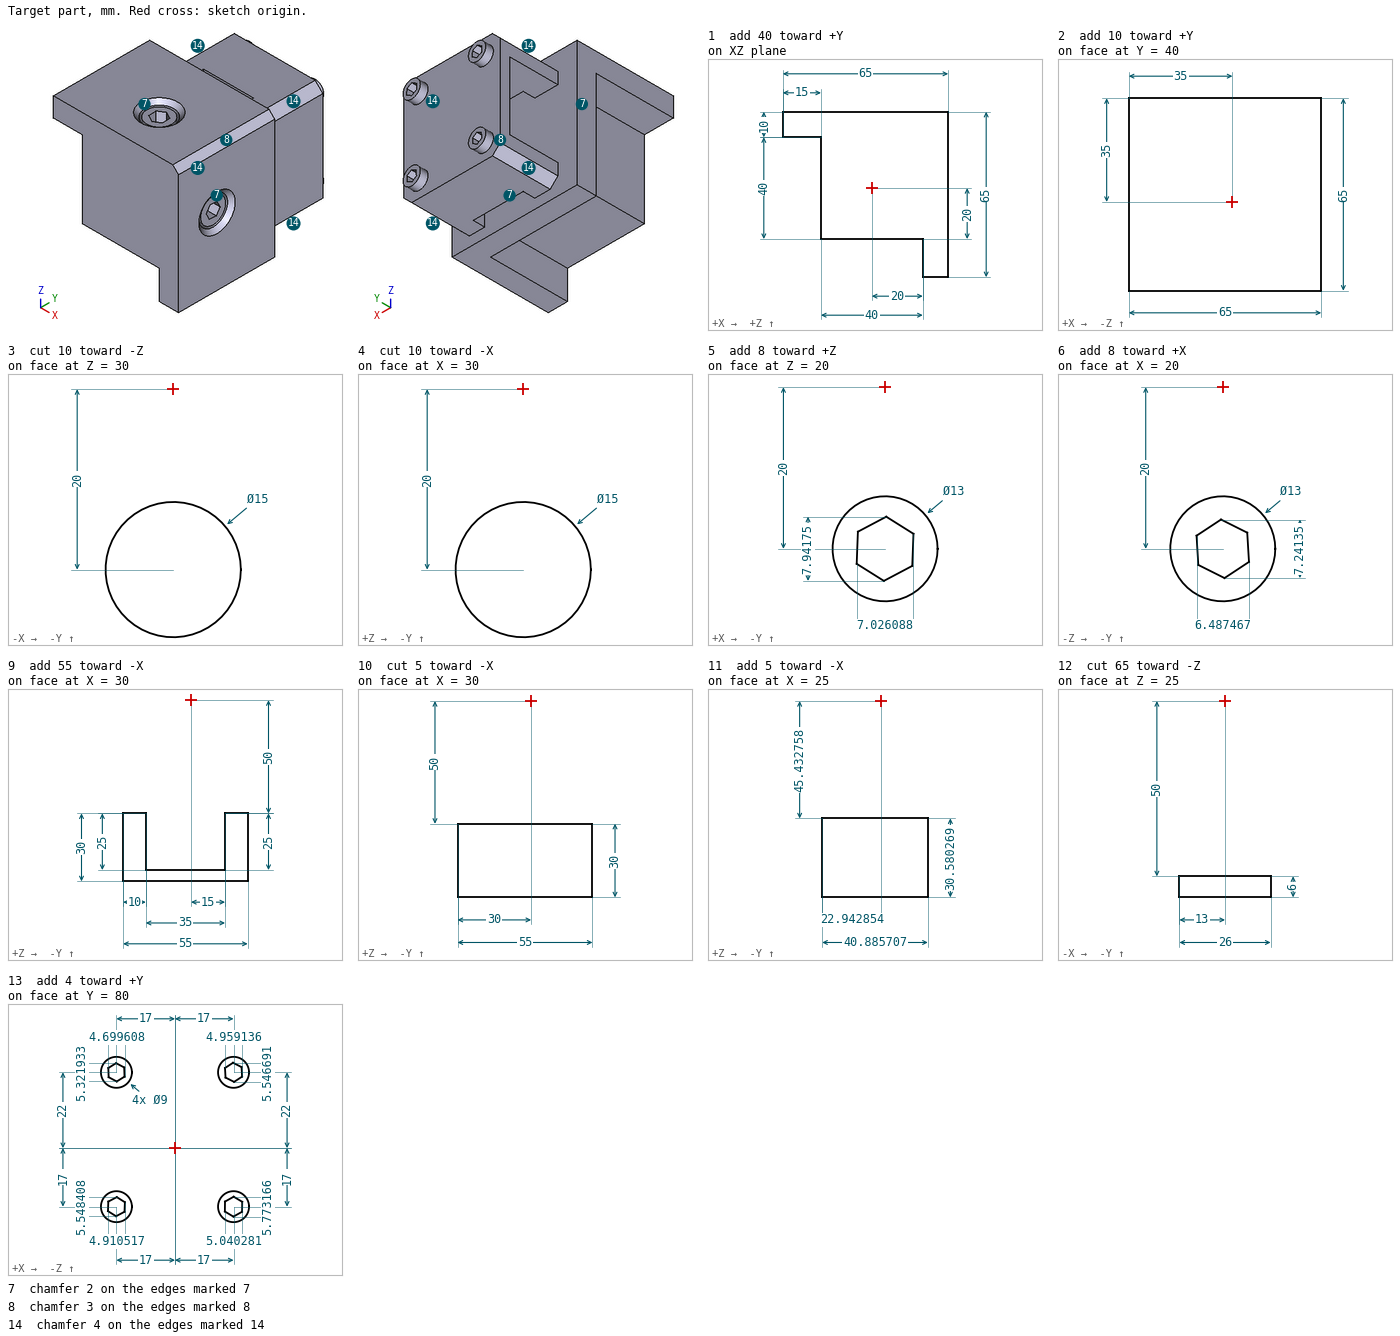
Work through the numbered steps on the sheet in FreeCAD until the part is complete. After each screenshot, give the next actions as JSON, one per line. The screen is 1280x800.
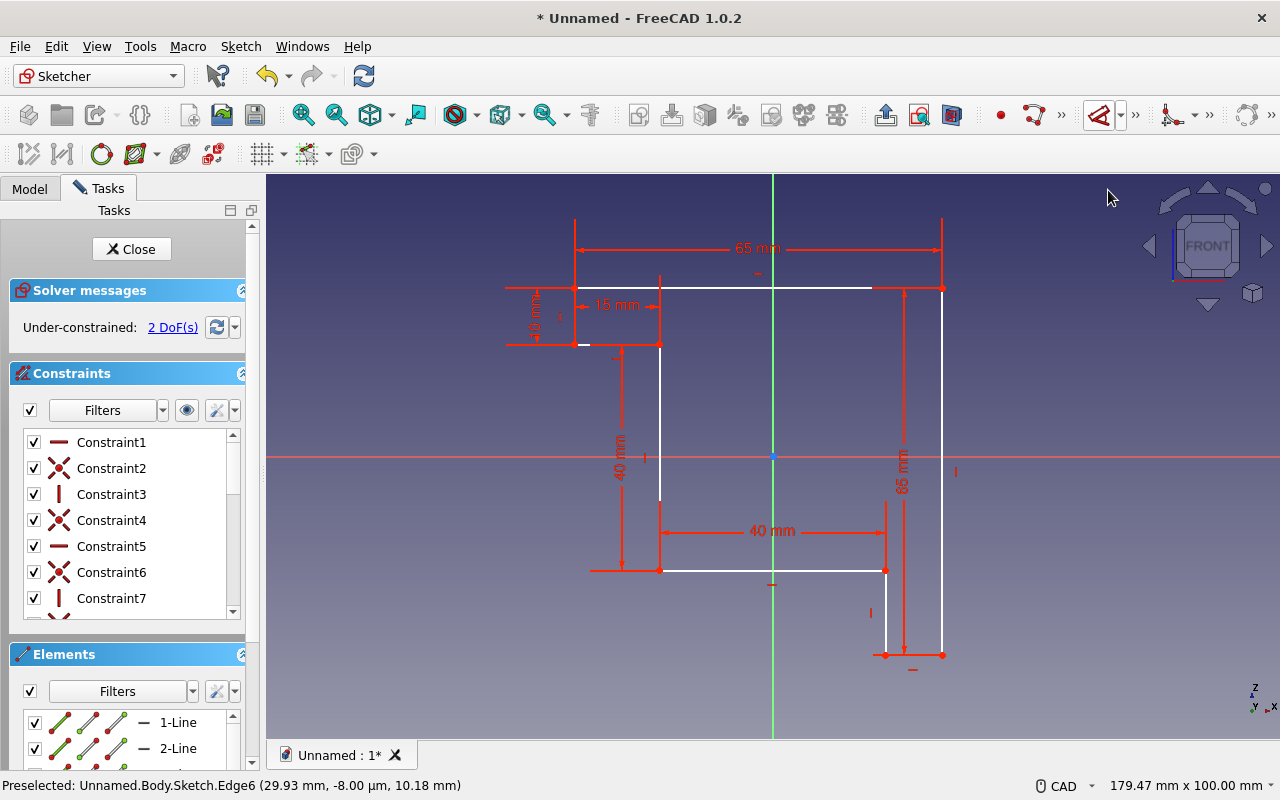
{"action": "left_click", "coordinate": [886, 571]}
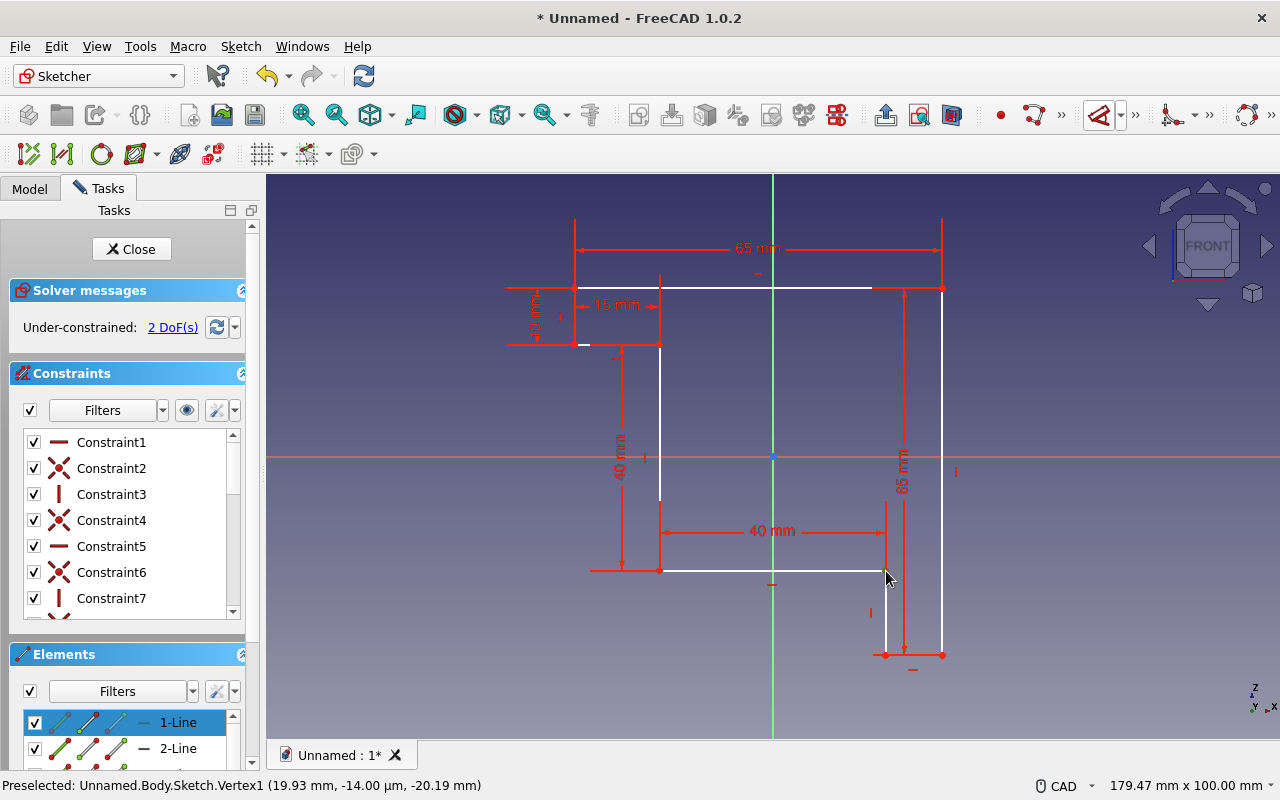
{"action": "key", "text": "l"}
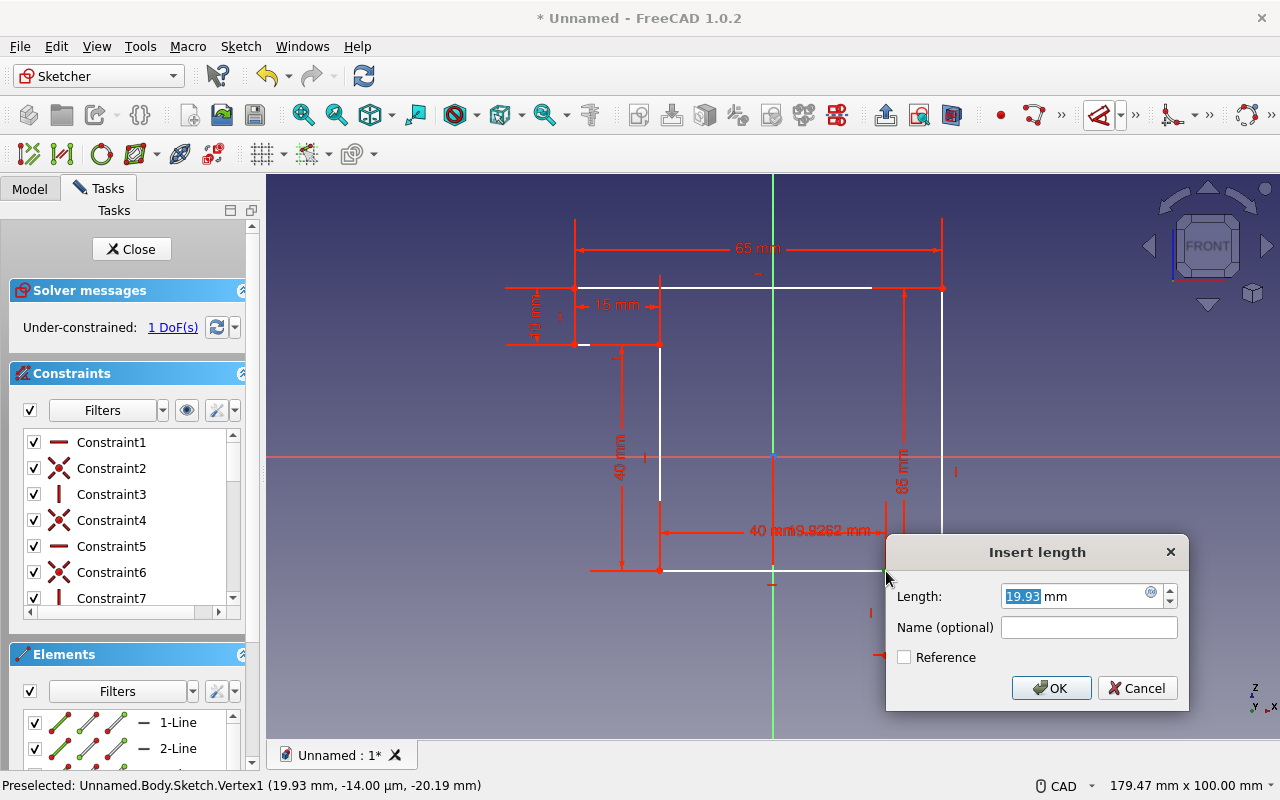
{"action": "type", "text": "20"}
{"action": "key", "text": "Return"}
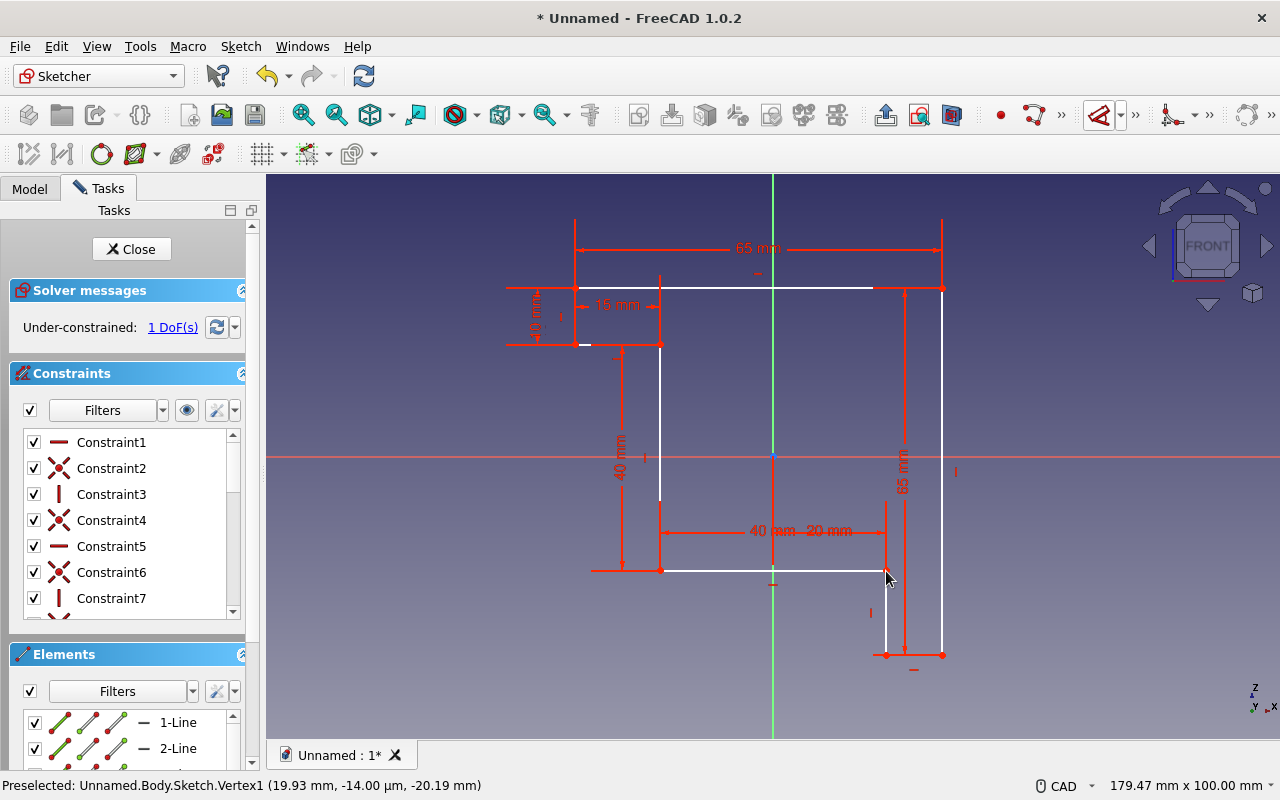
{"action": "left_click", "coordinate": [886, 571]}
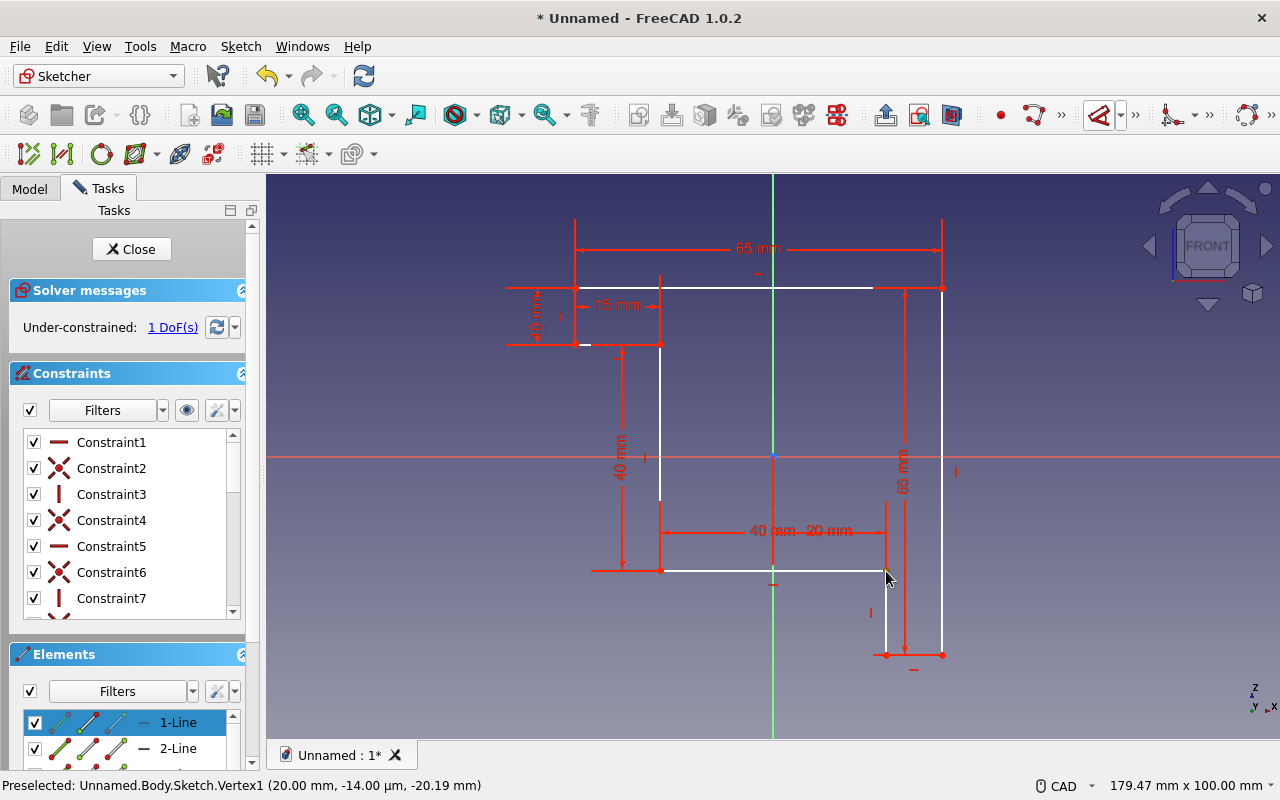
{"action": "key", "text": "i"}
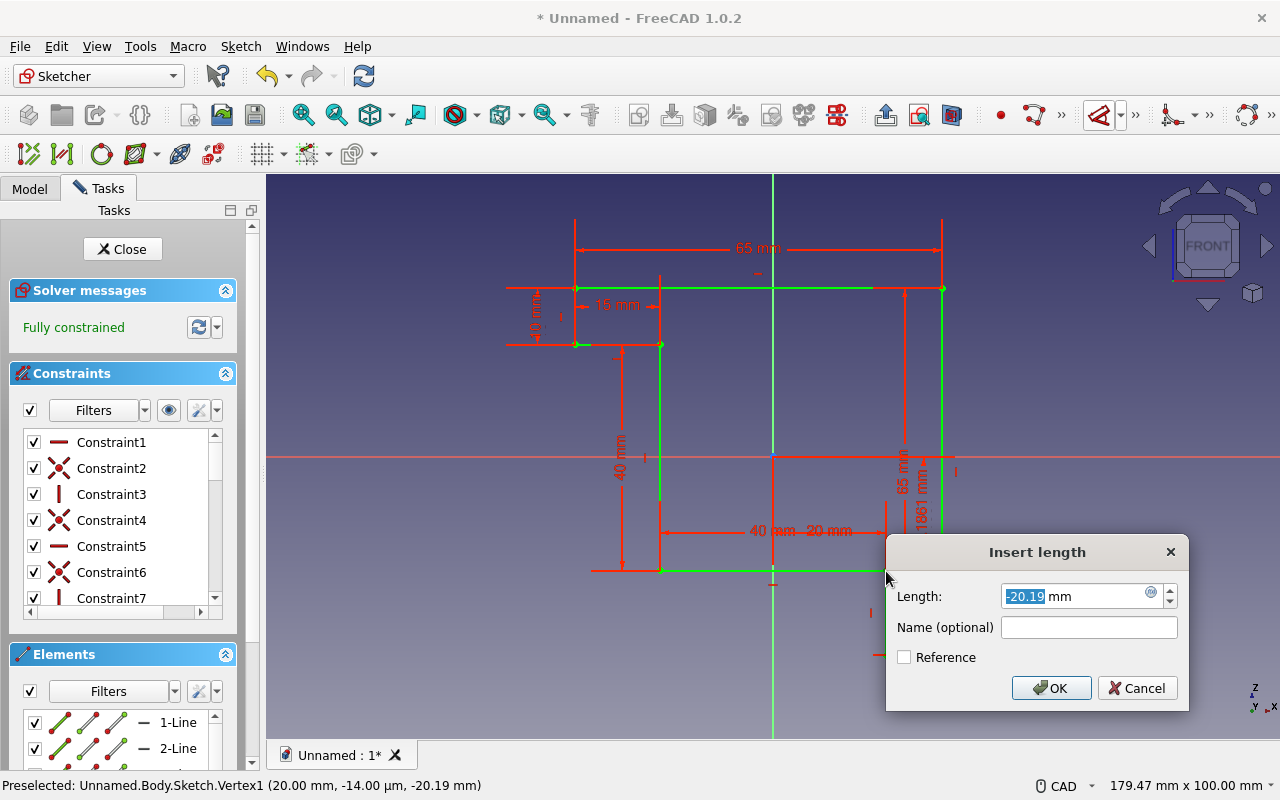
{"action": "type", "text": "-20"}
{"action": "key", "text": "Return"}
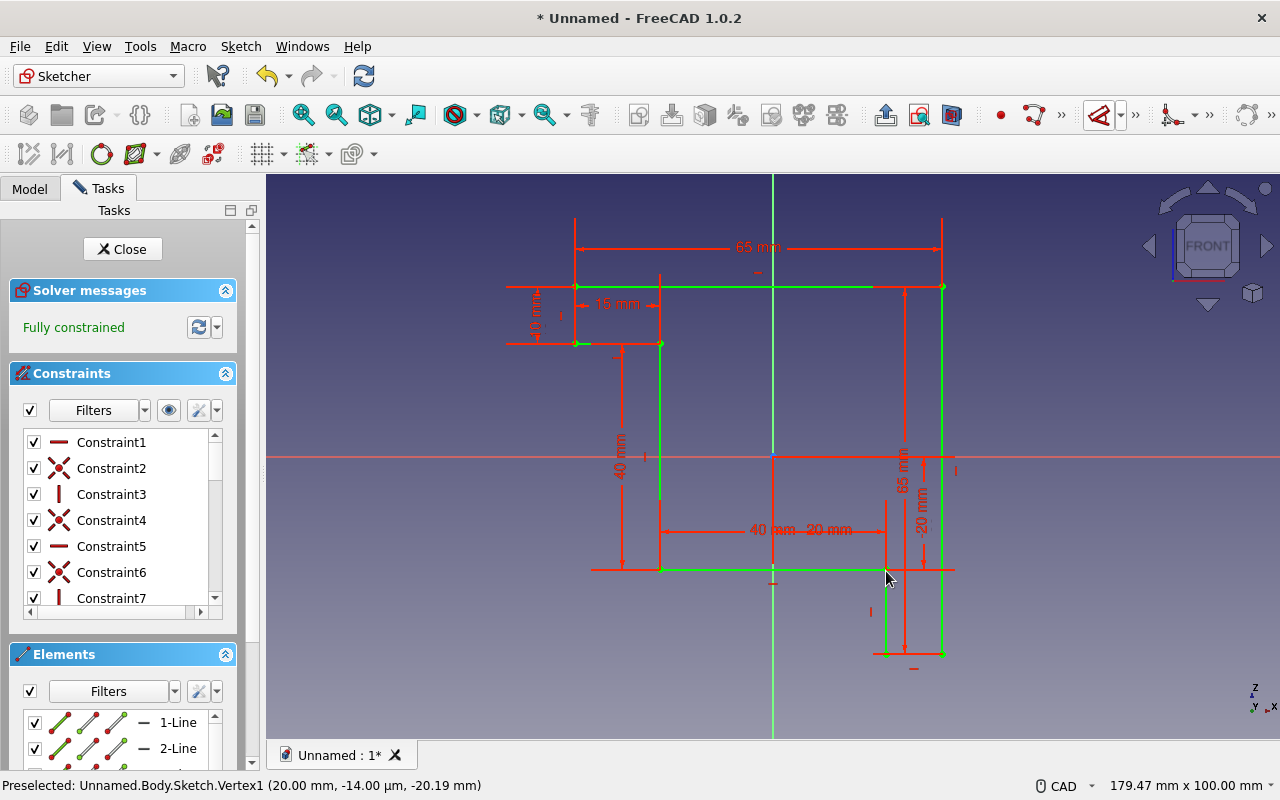
{"action": "left_click", "coordinate": [123, 249]}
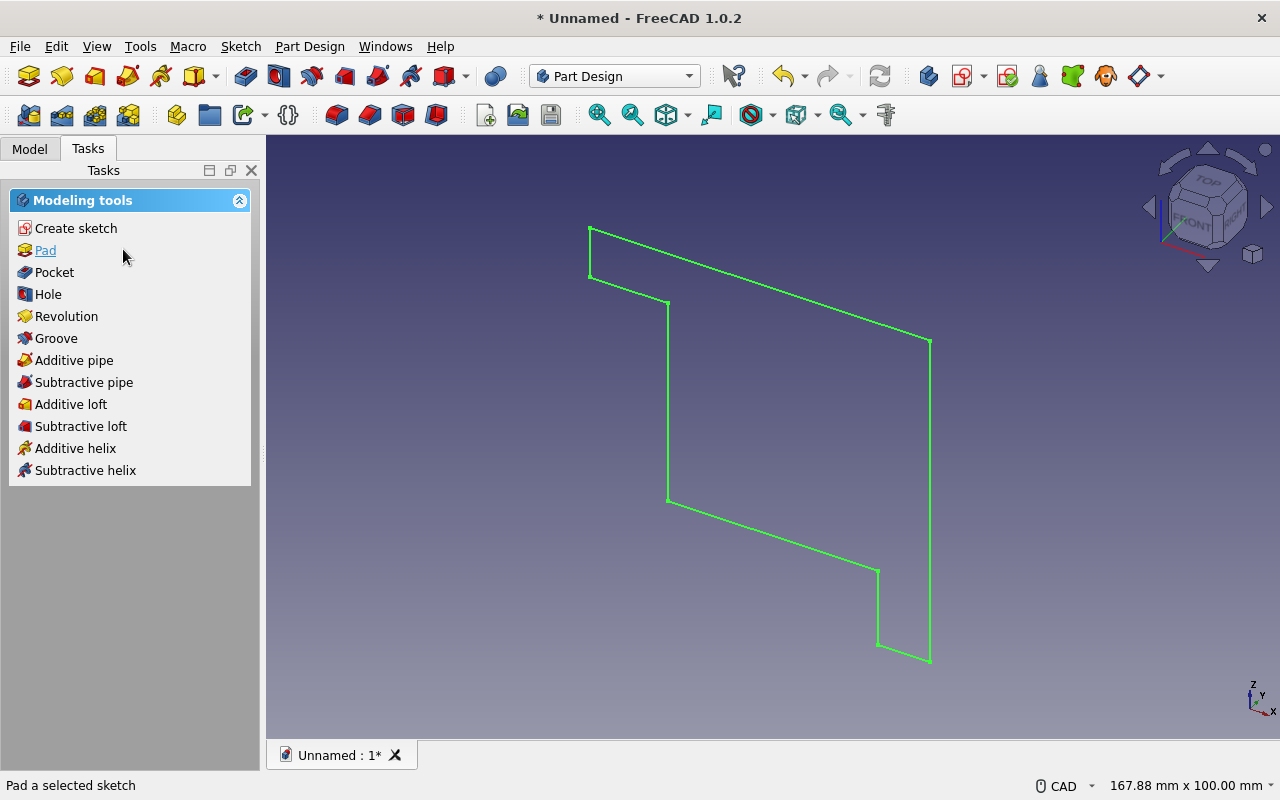
{"action": "left_click", "coordinate": [29, 76]}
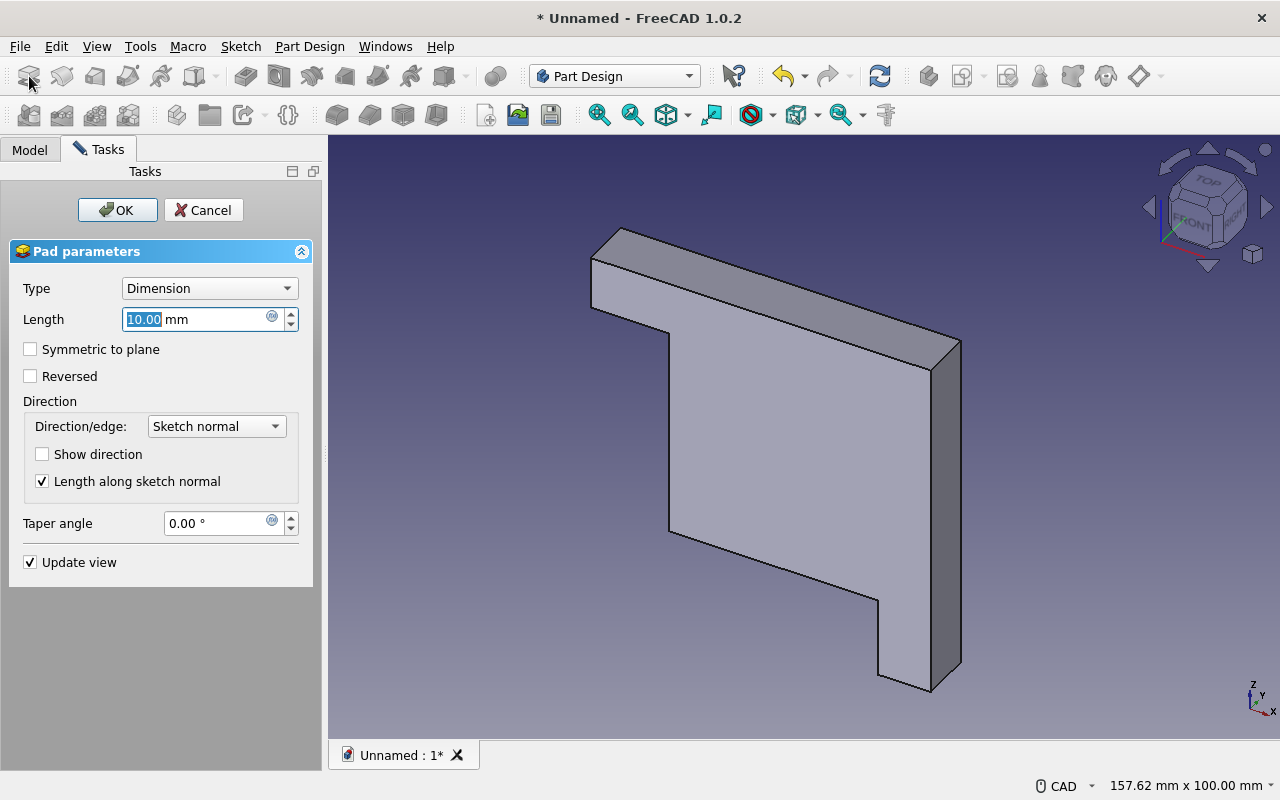
{"action": "type", "text": "40"}
{"action": "key", "text": "Tab"}